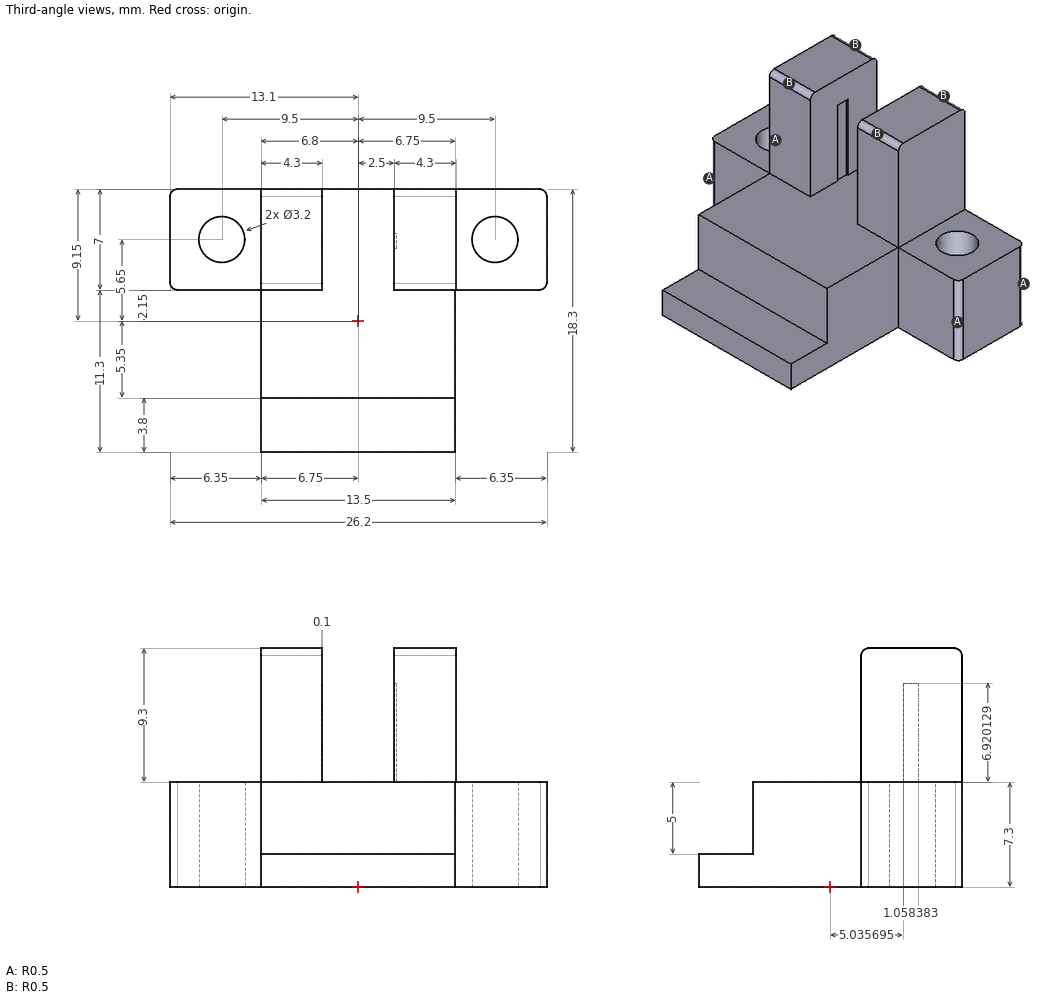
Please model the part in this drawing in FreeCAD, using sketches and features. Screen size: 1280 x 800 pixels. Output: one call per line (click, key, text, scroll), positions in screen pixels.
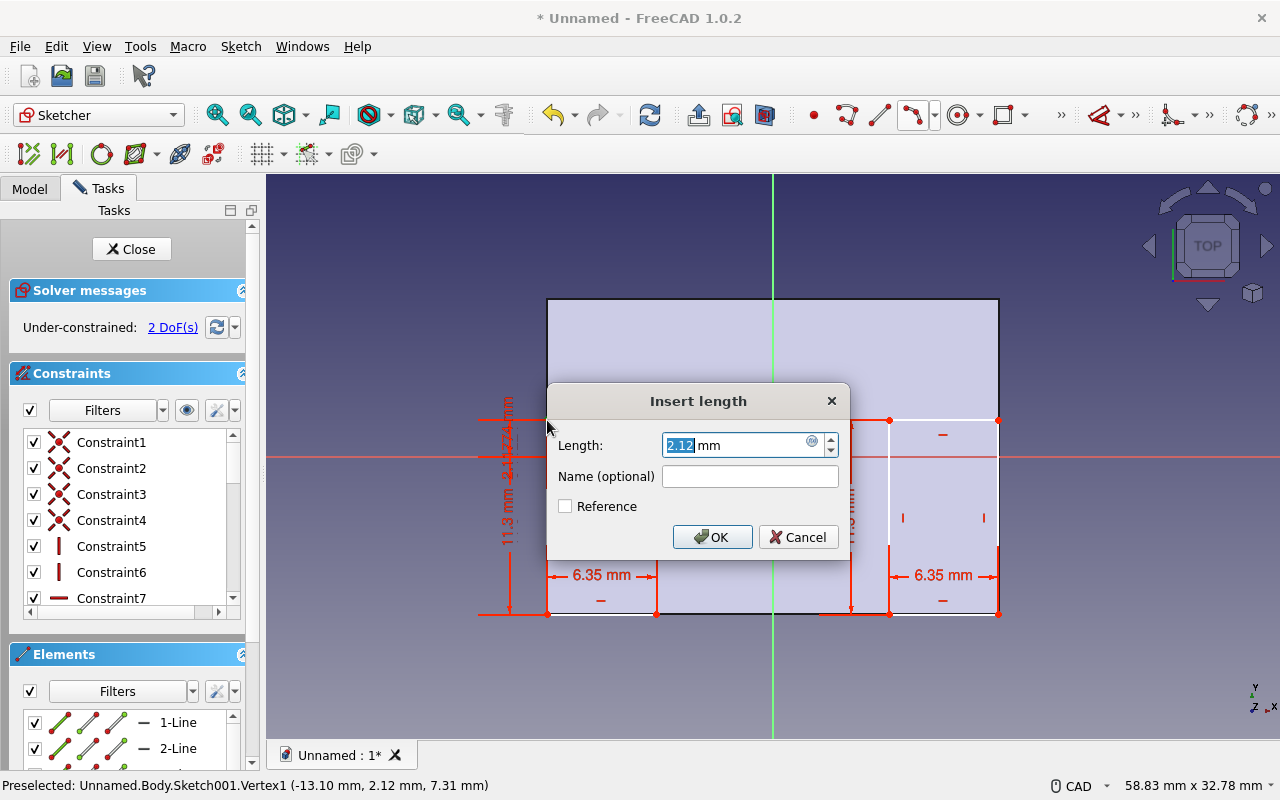
text(2.15)
key(Return)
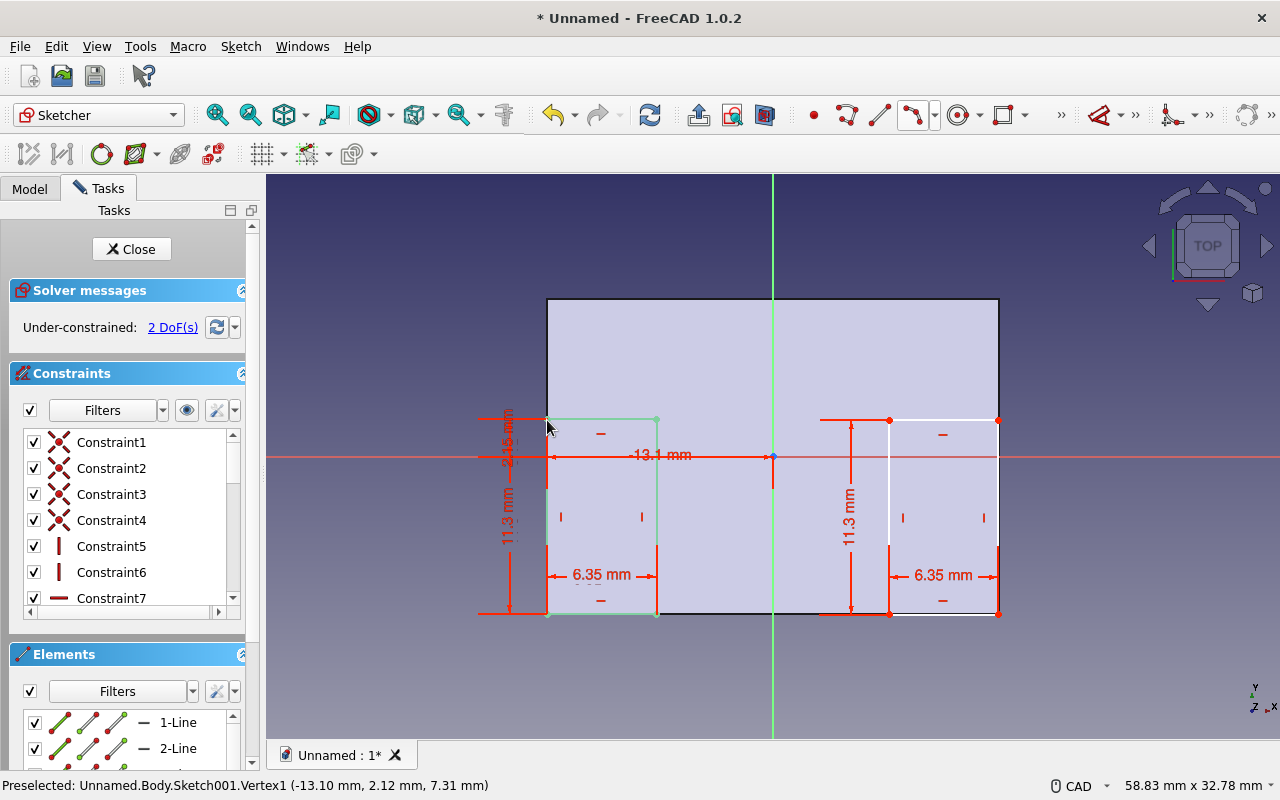
click(889, 420)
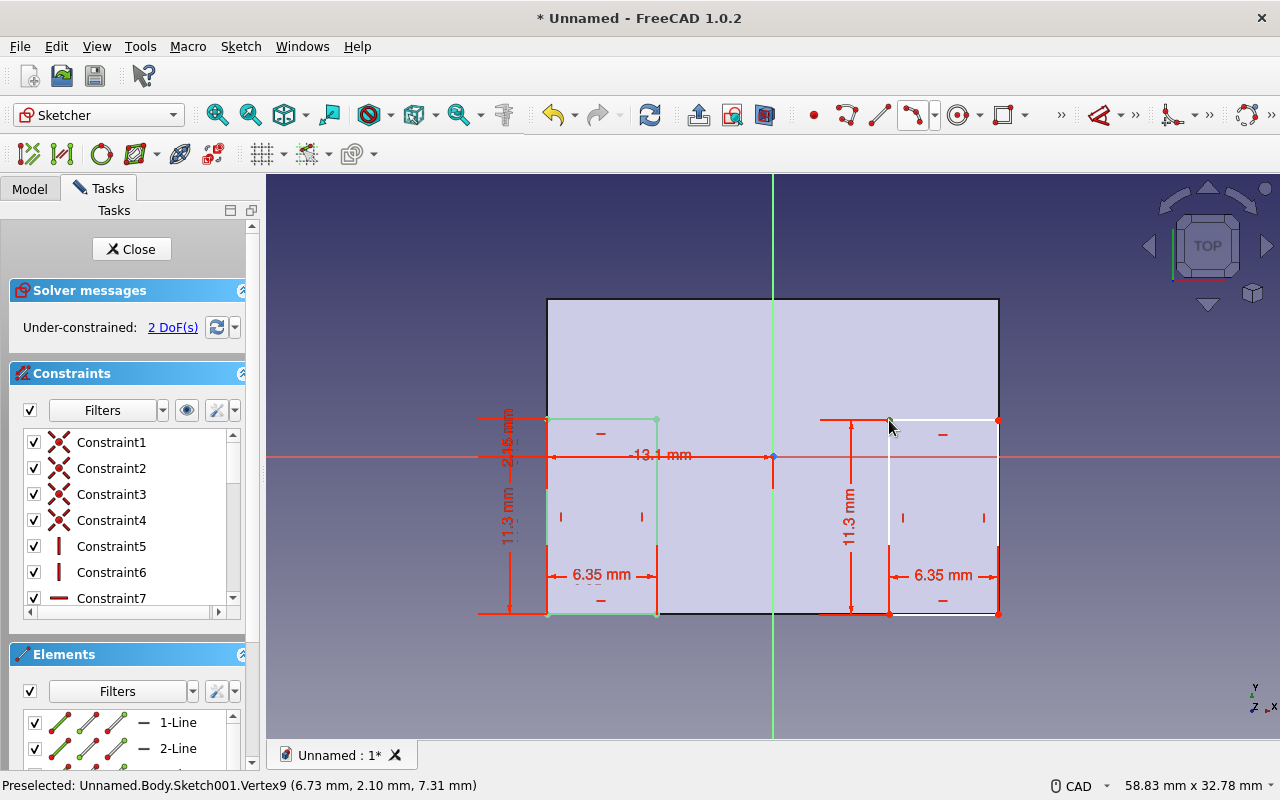
click(1120, 116)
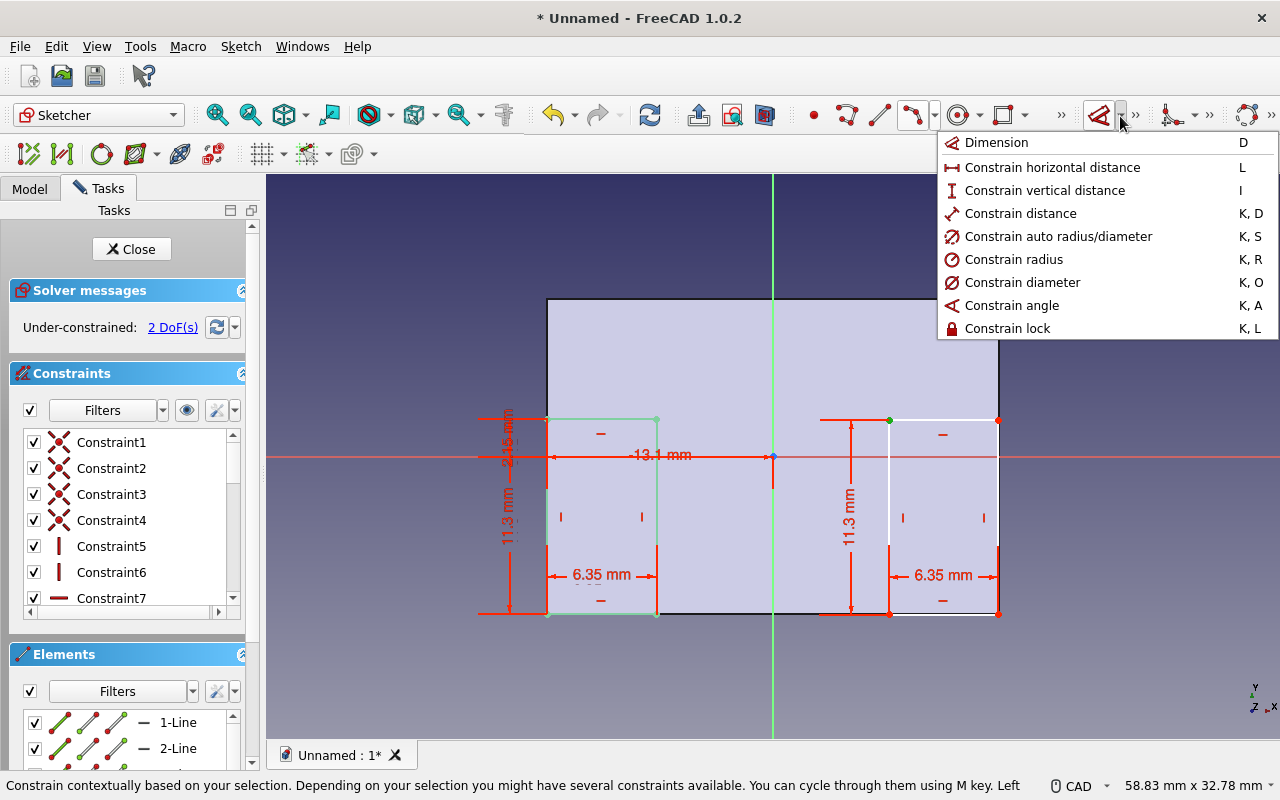
click(1108, 168)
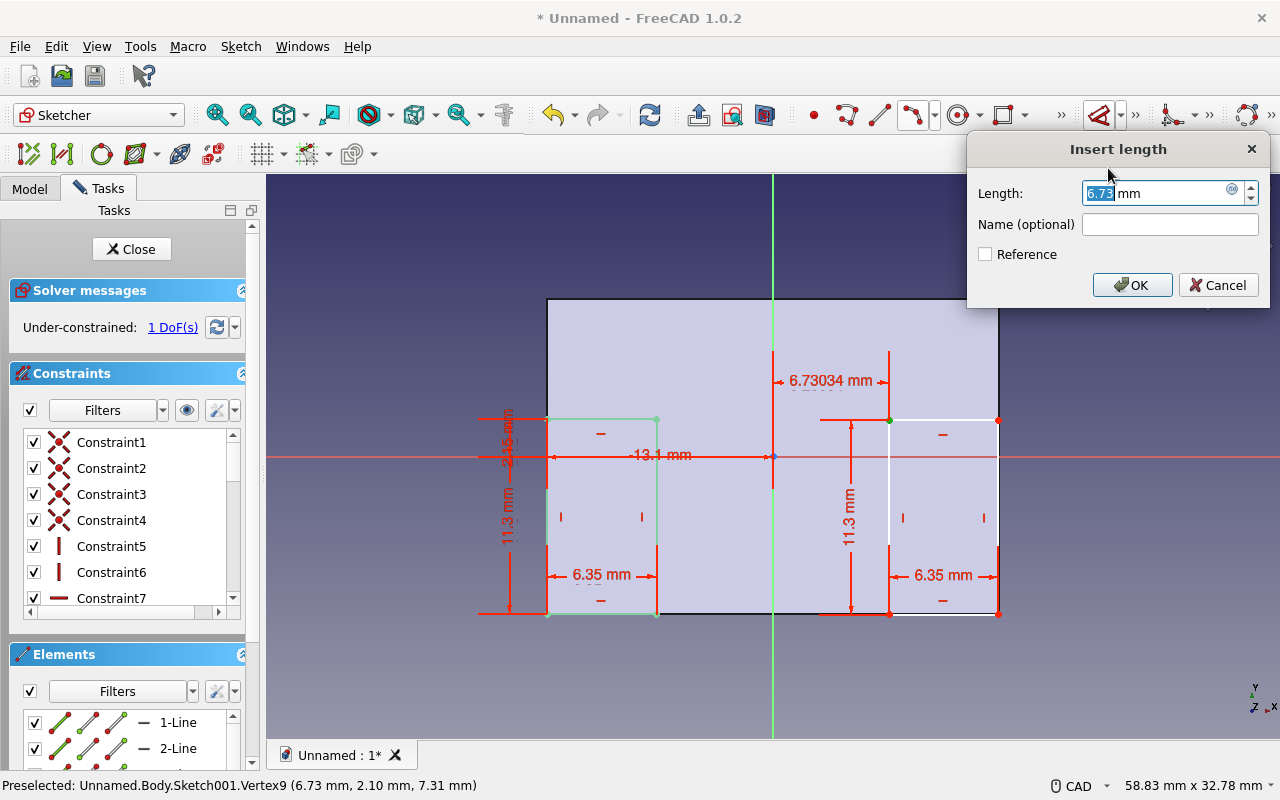
text(6.75)
key(Return)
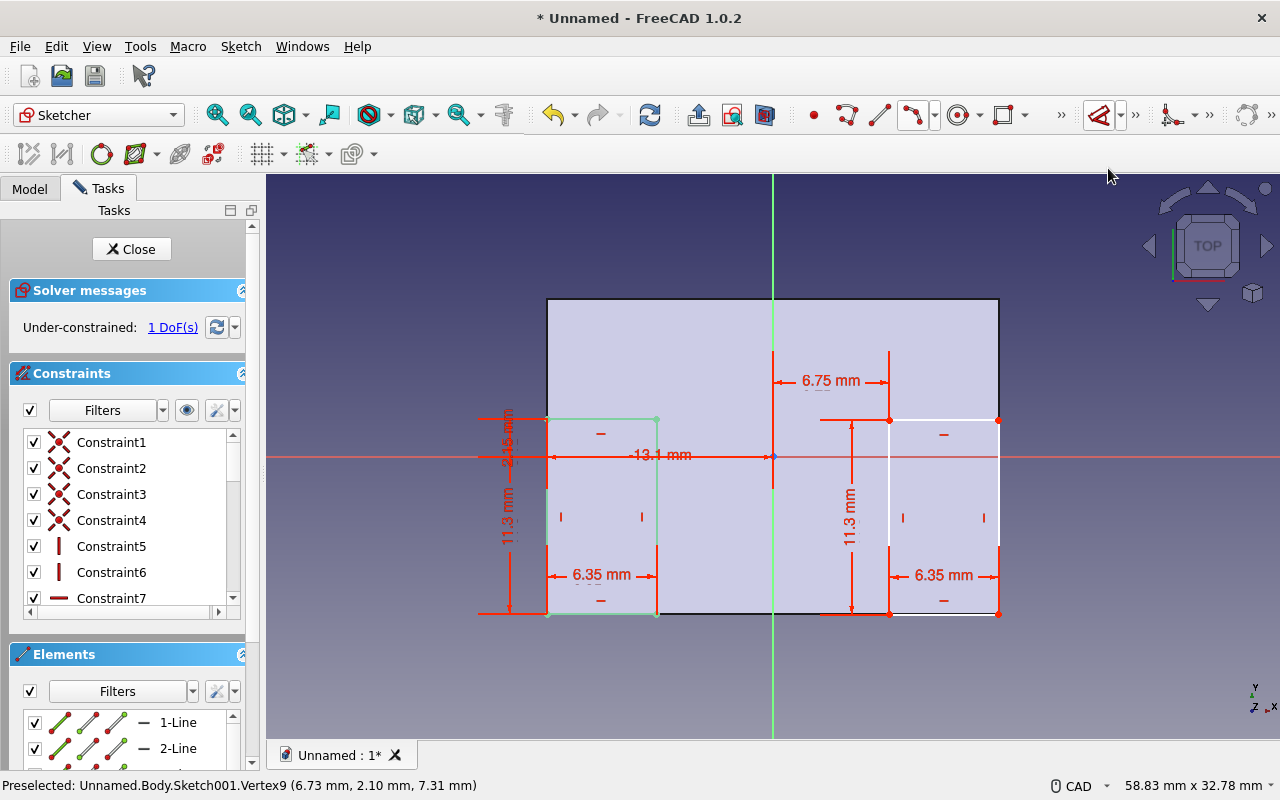
click(889, 420)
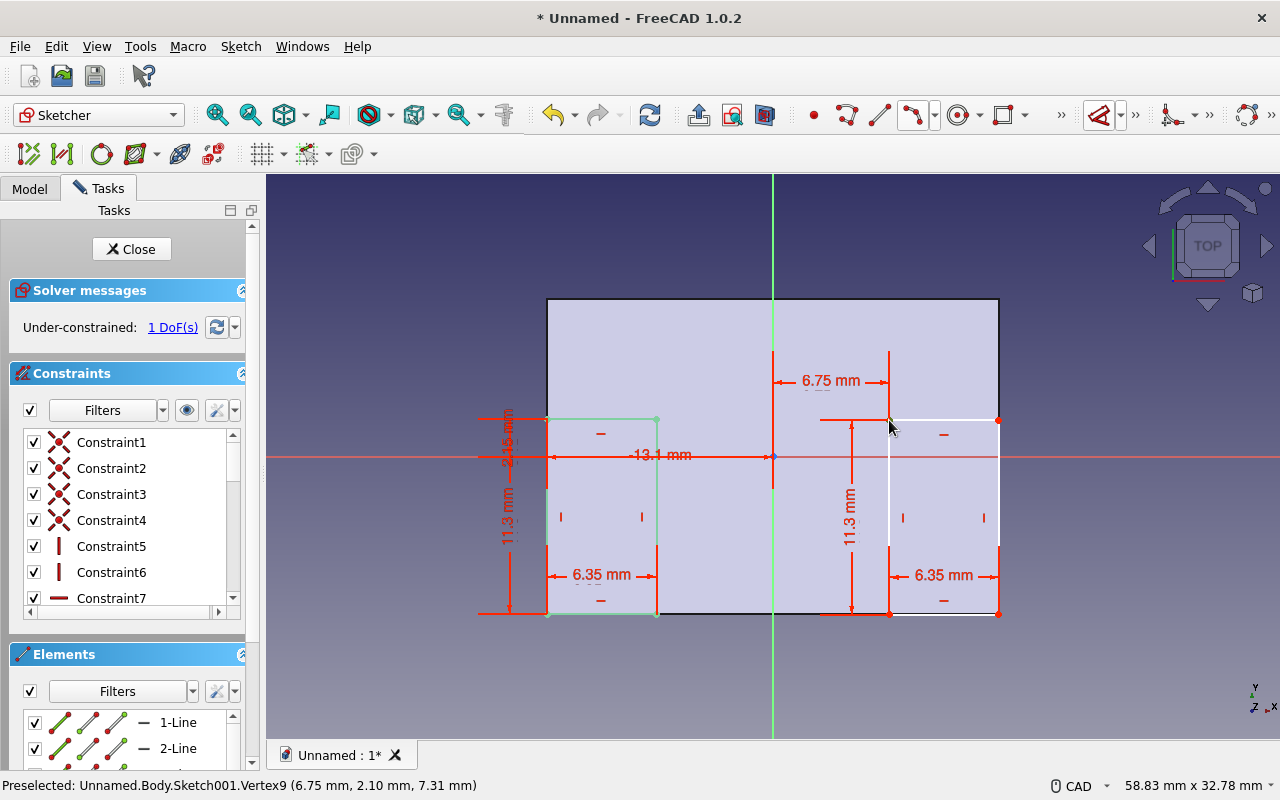
key(i)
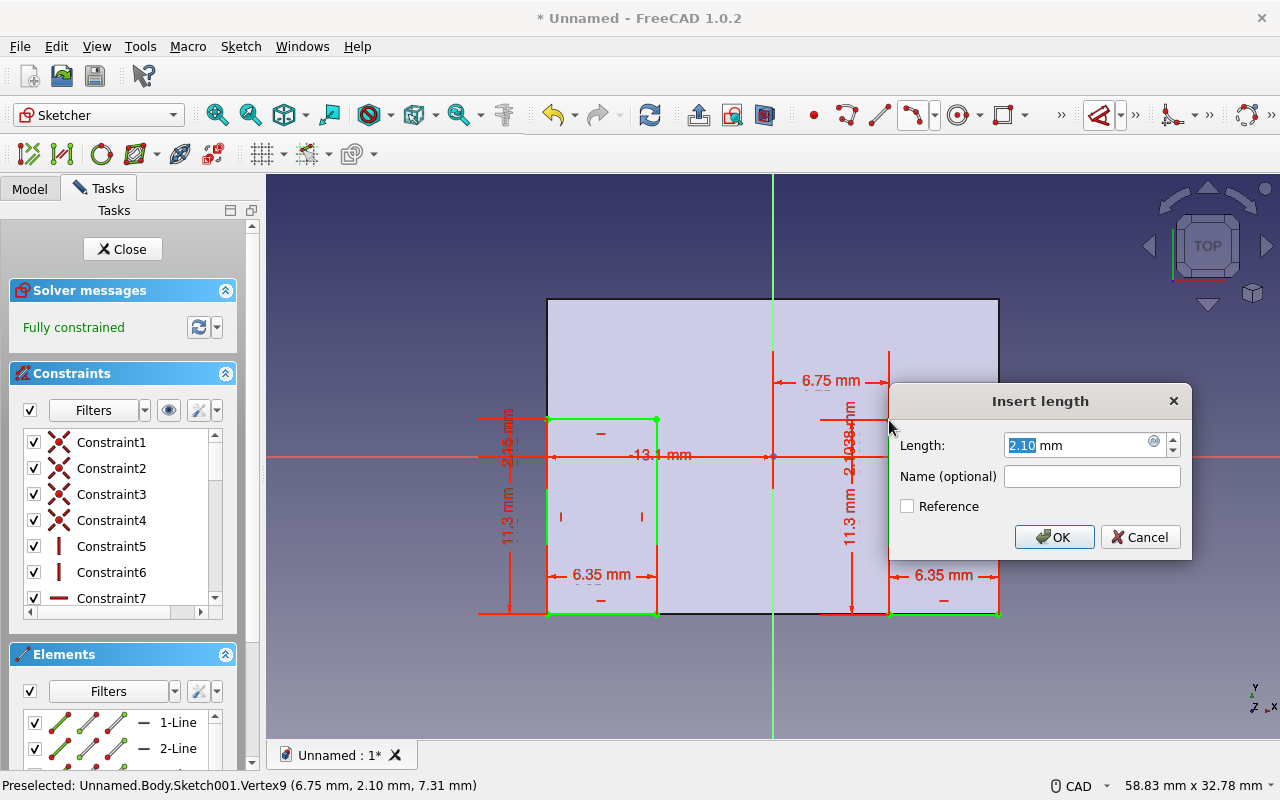
text(2.15)
key(Return)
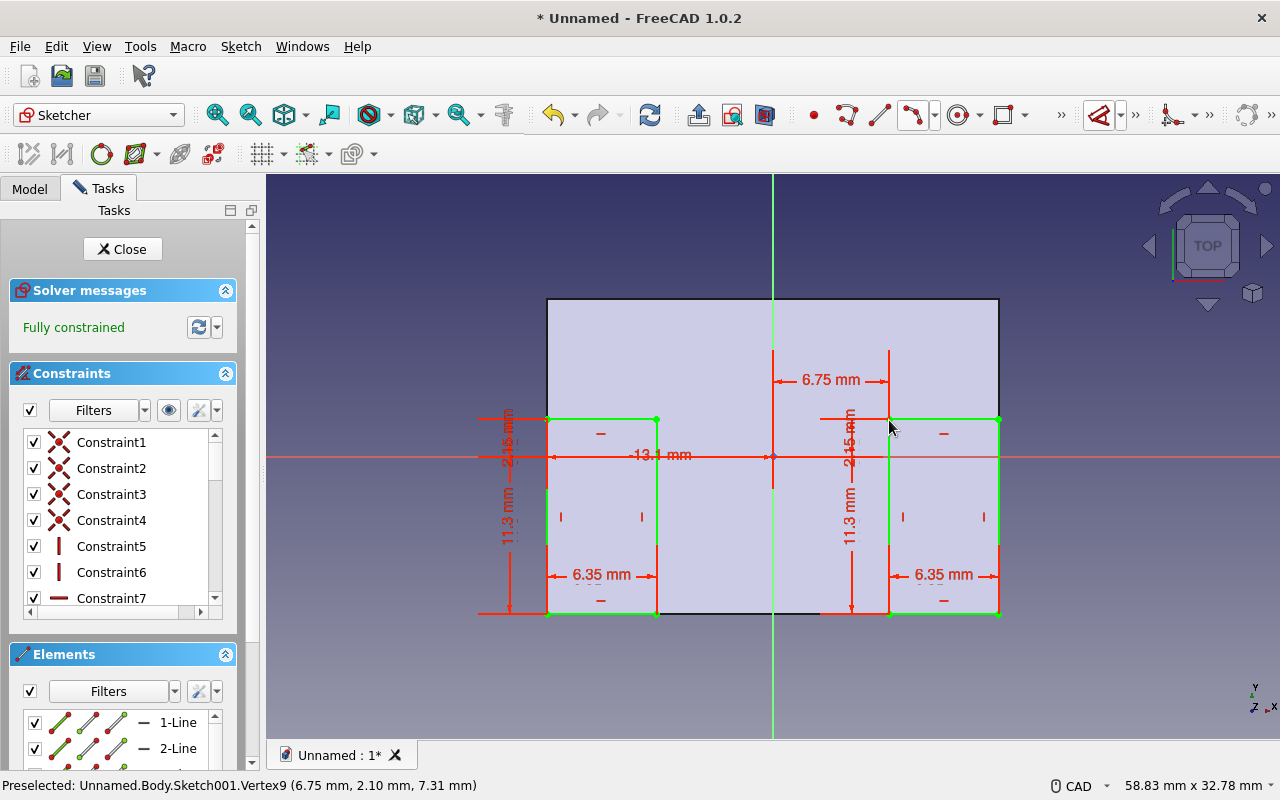
click(123, 249)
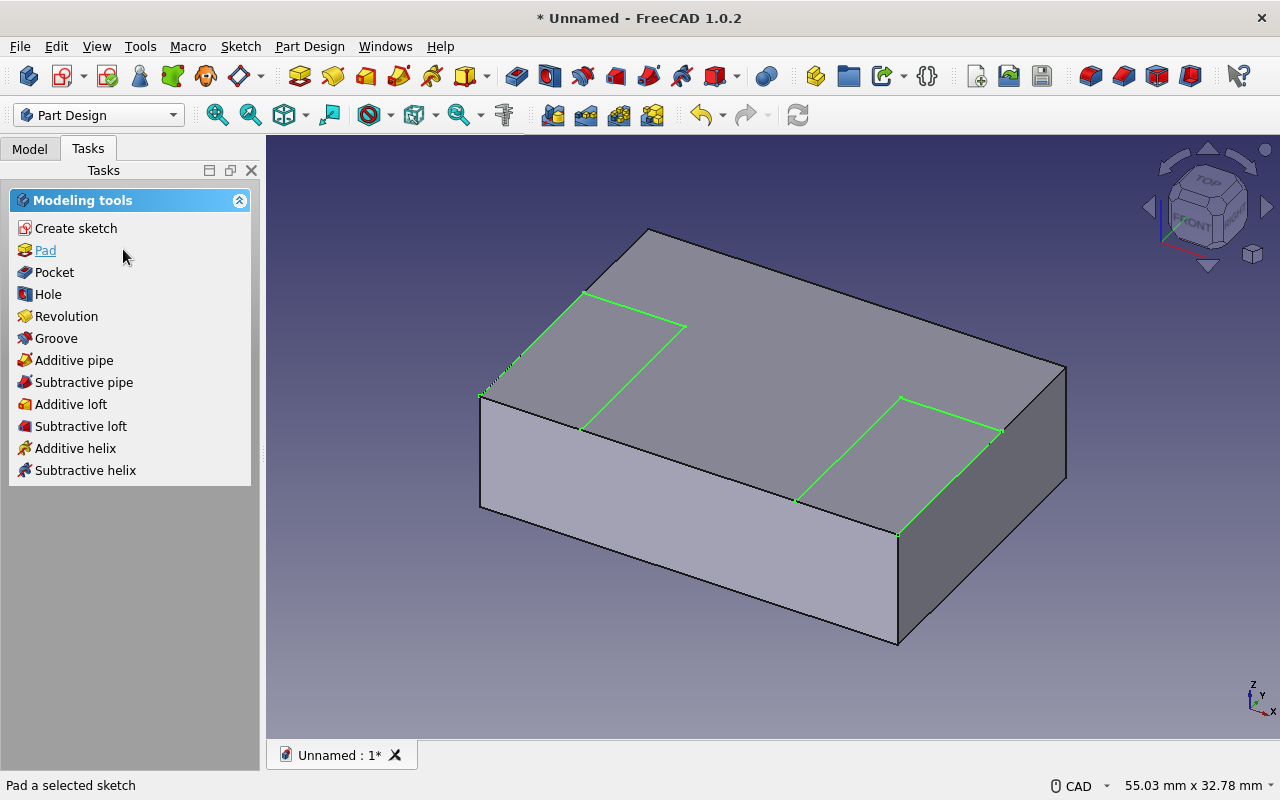
click(517, 76)